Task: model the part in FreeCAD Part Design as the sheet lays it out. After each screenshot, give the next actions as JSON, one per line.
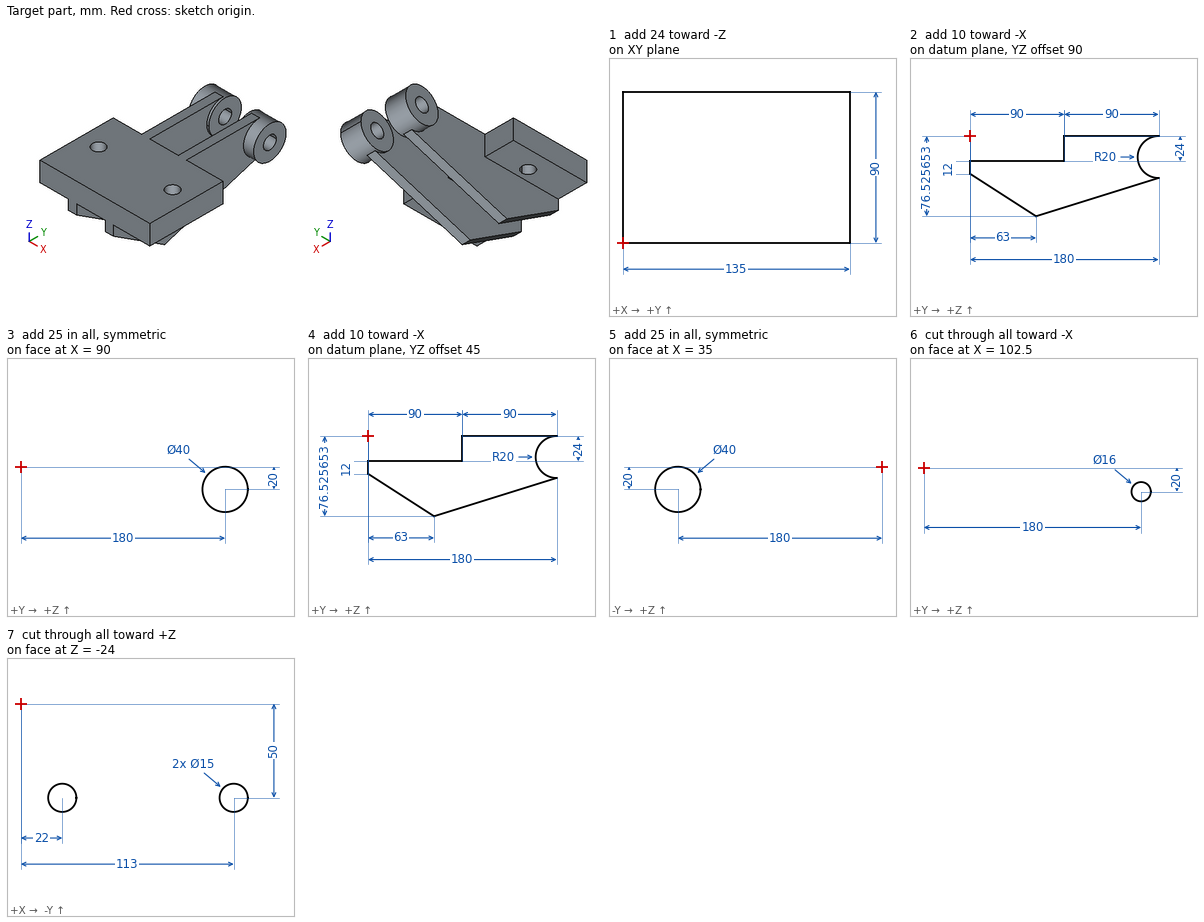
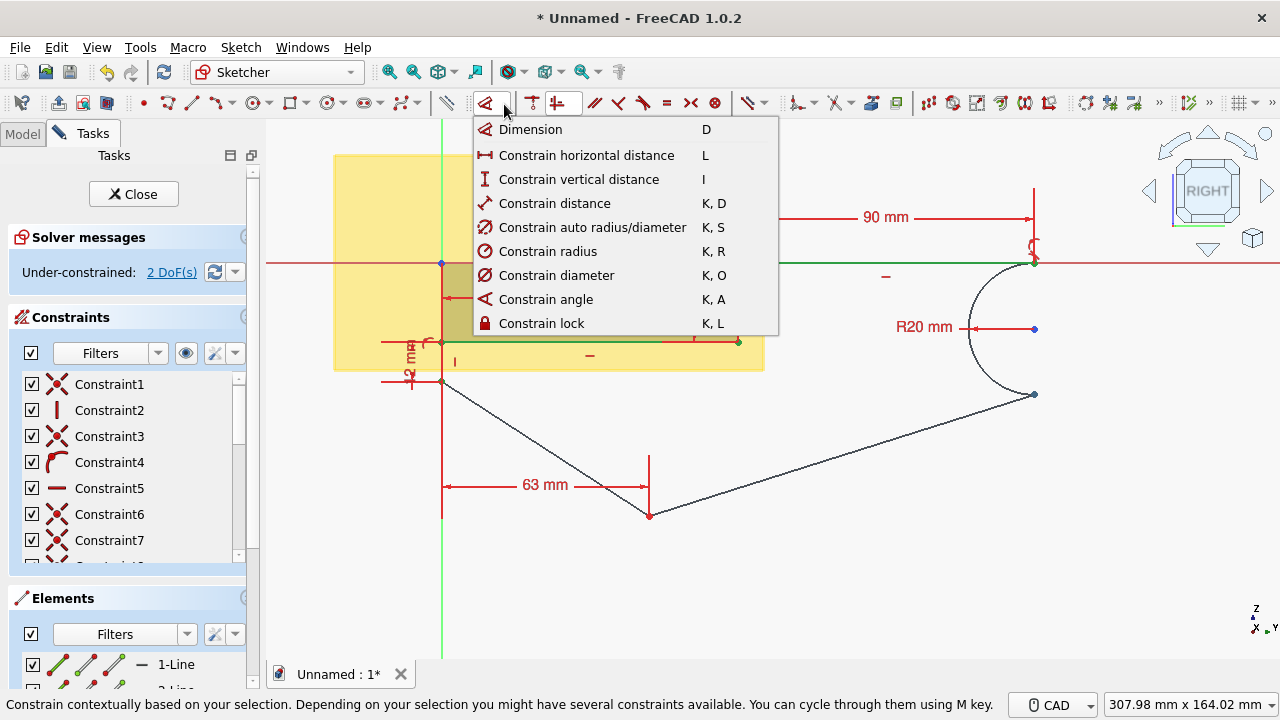
{"action": "left_click", "coordinate": [626, 155]}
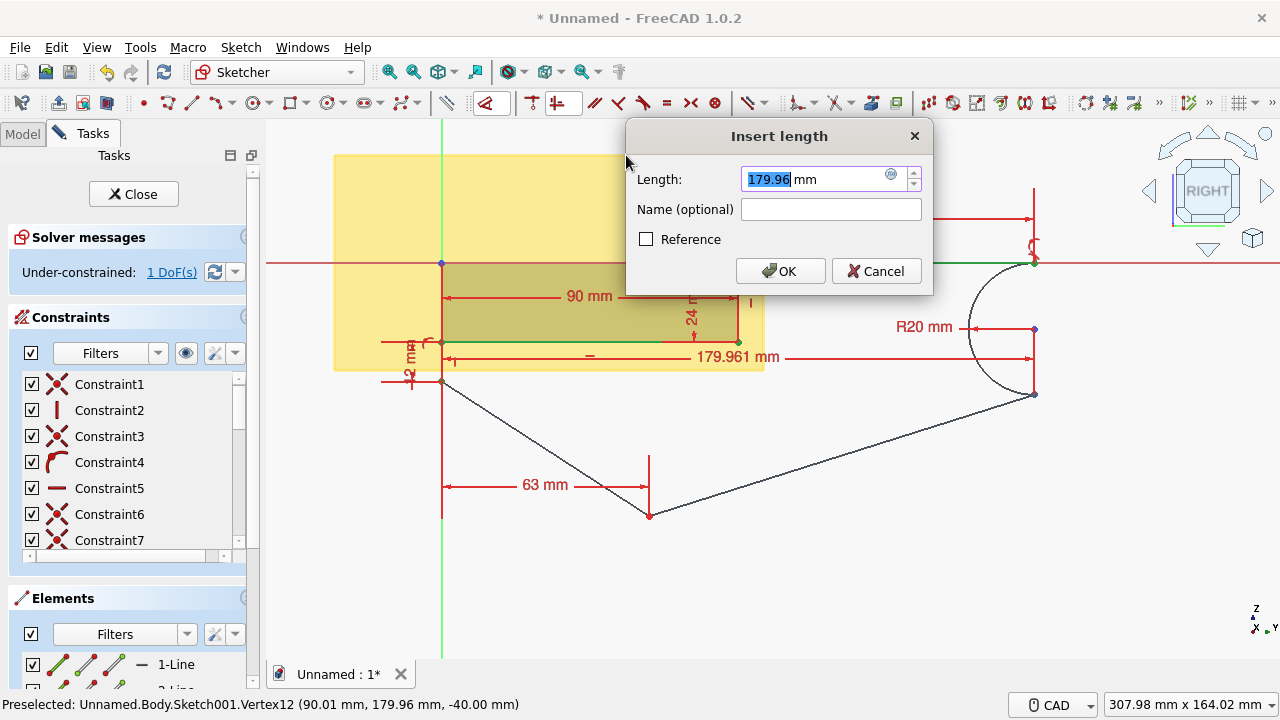
{"action": "type", "text": "180"}
{"action": "key", "text": "Return"}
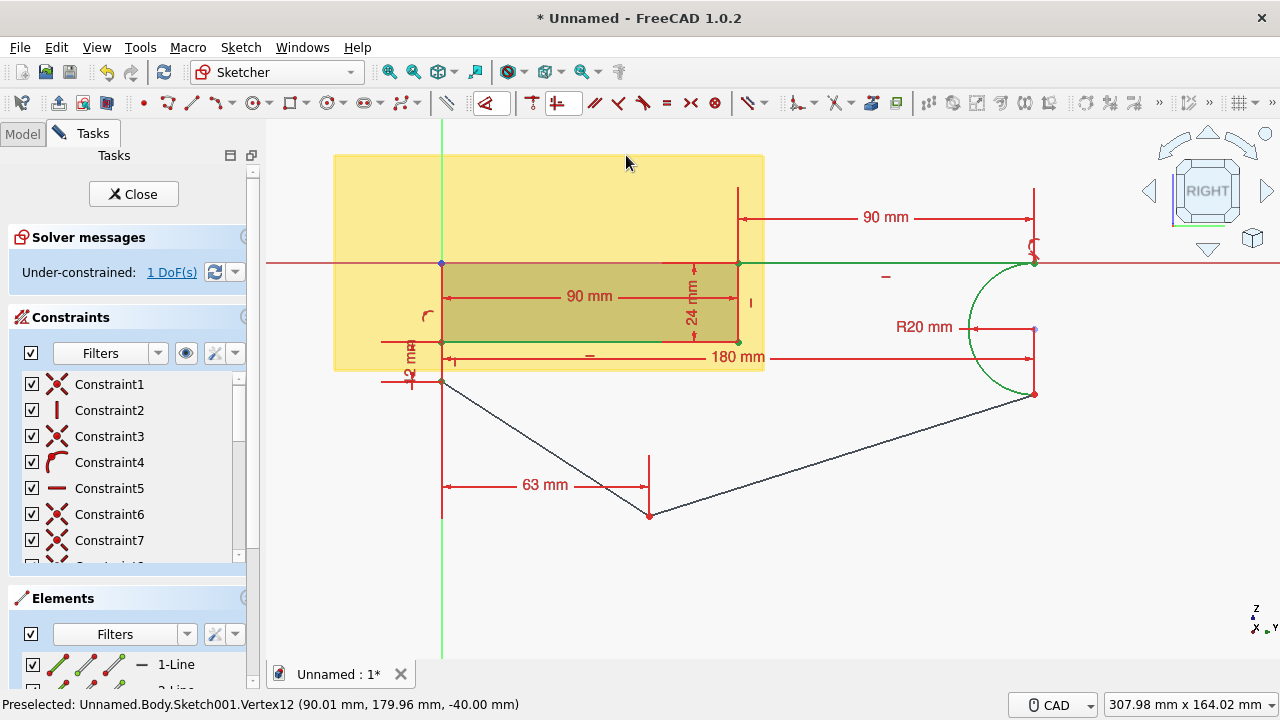
{"action": "left_click", "coordinate": [649, 516]}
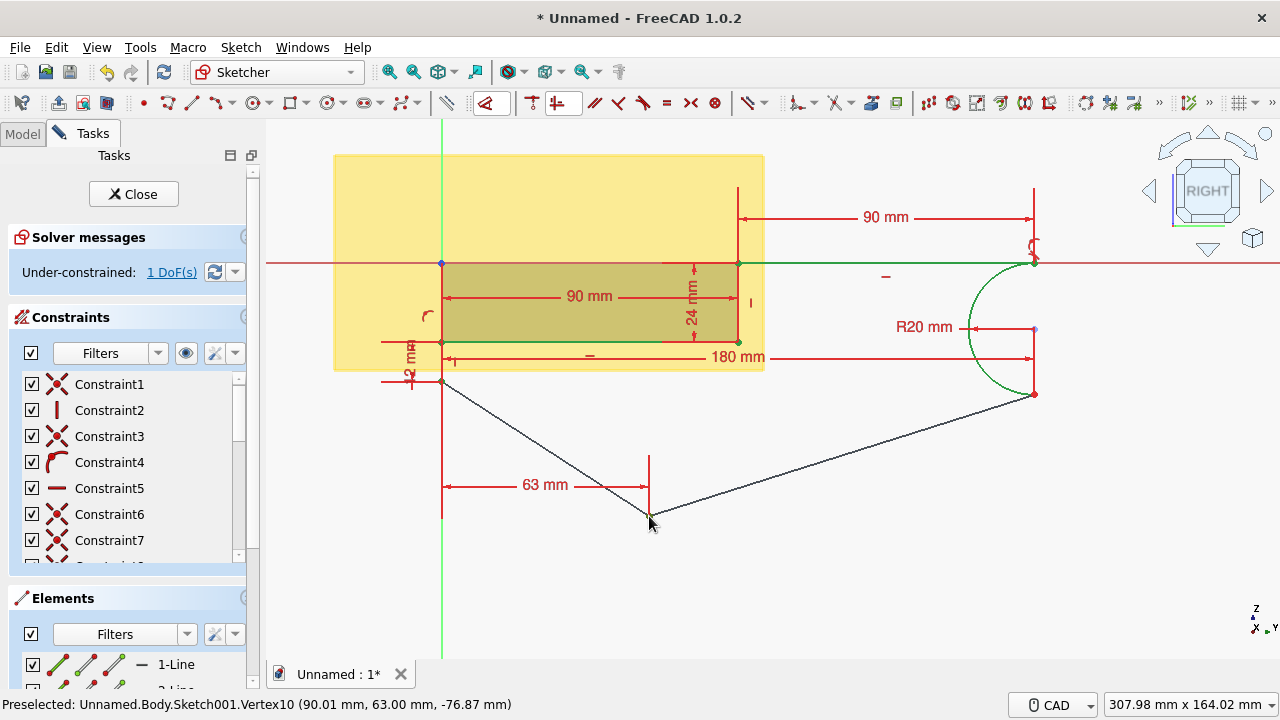
{"action": "left_click", "coordinate": [504, 104]}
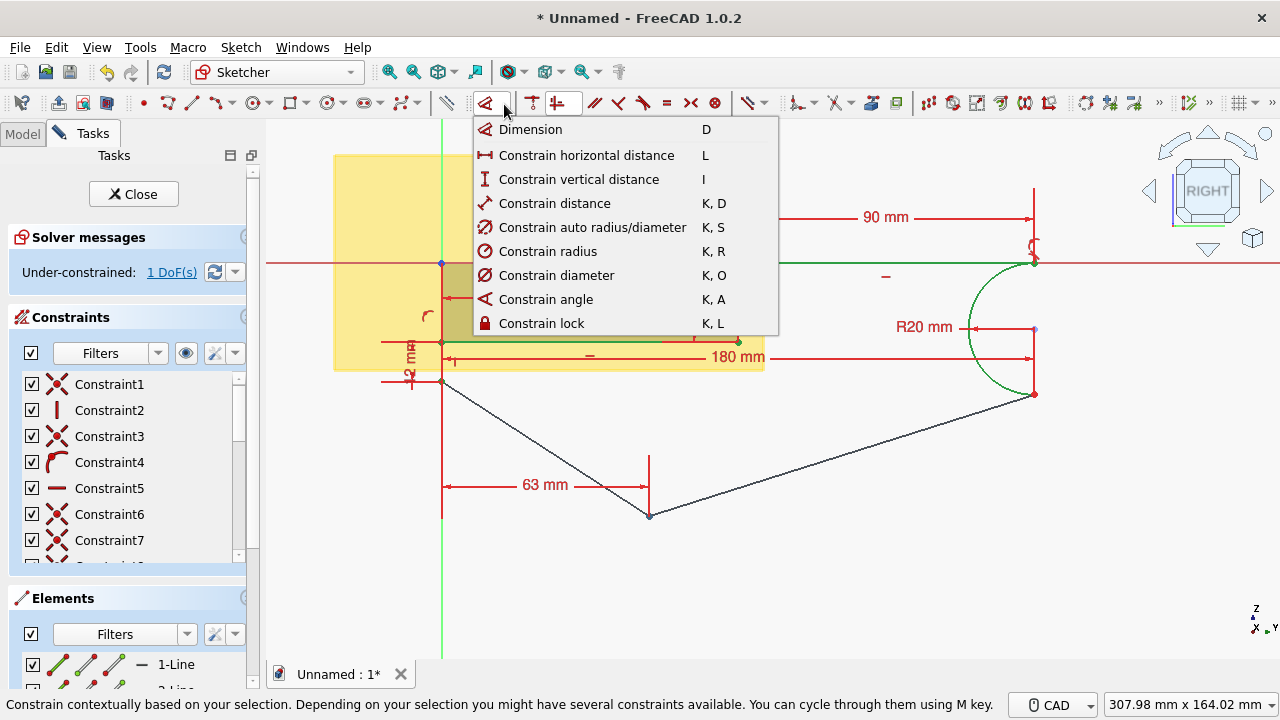
{"action": "left_click", "coordinate": [626, 179]}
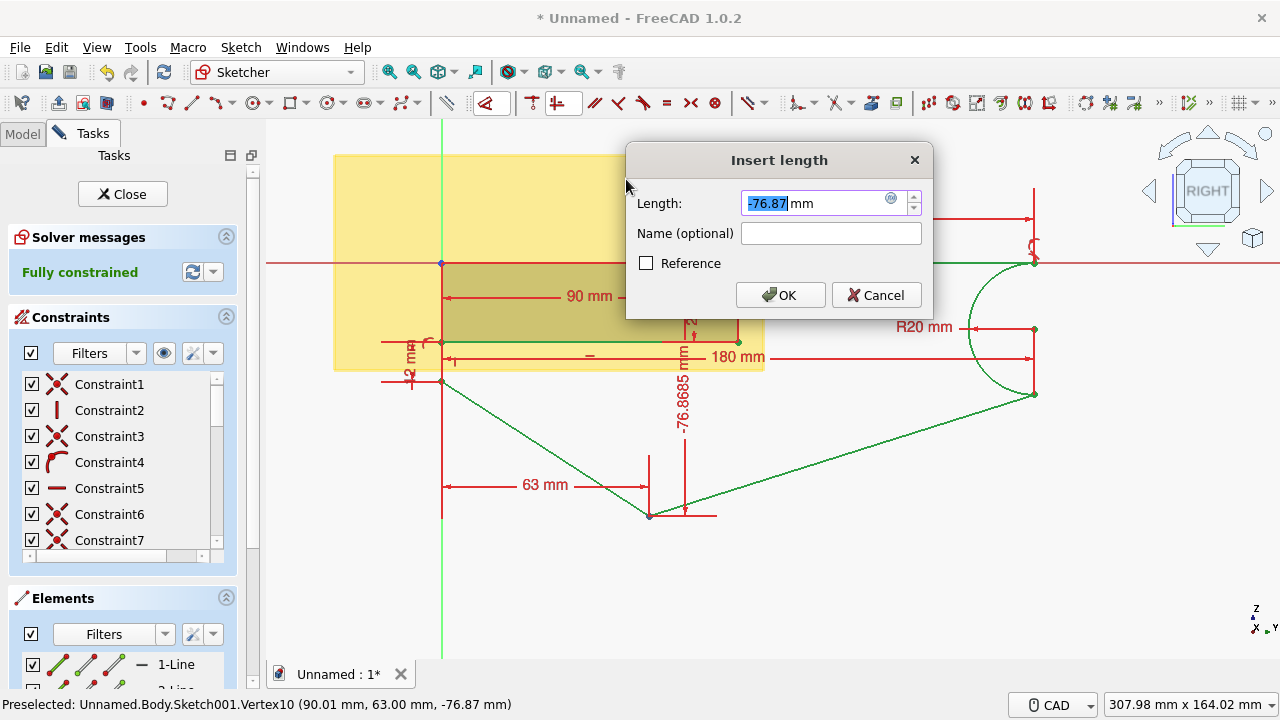
{"action": "type", "text": "-76.525653"}
{"action": "key", "text": "Return"}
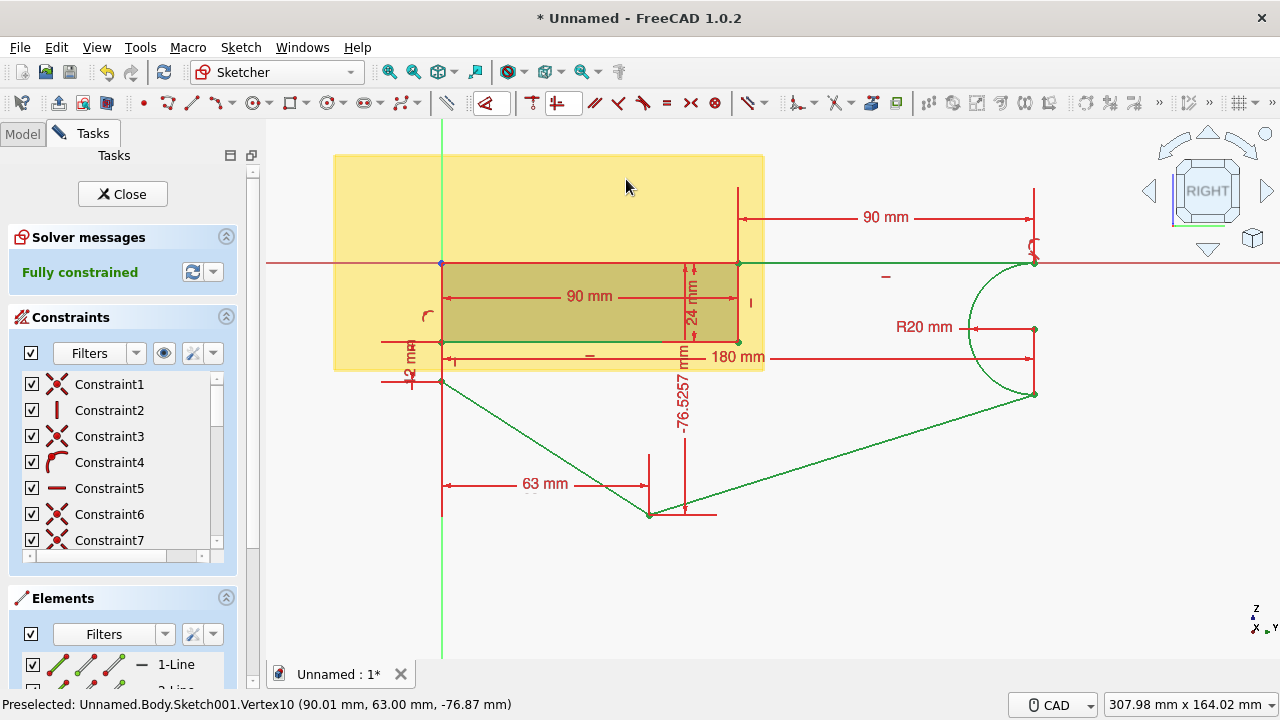
{"action": "left_click", "coordinate": [123, 194]}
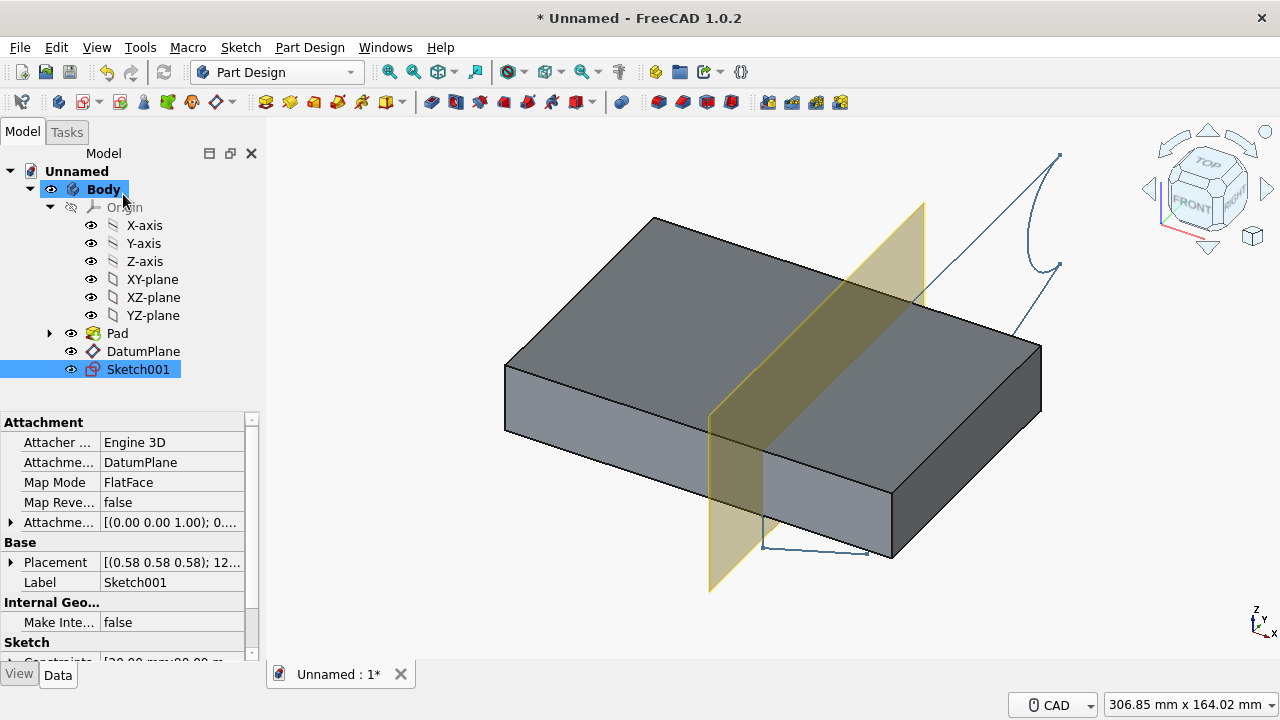
{"action": "left_click", "coordinate": [266, 102]}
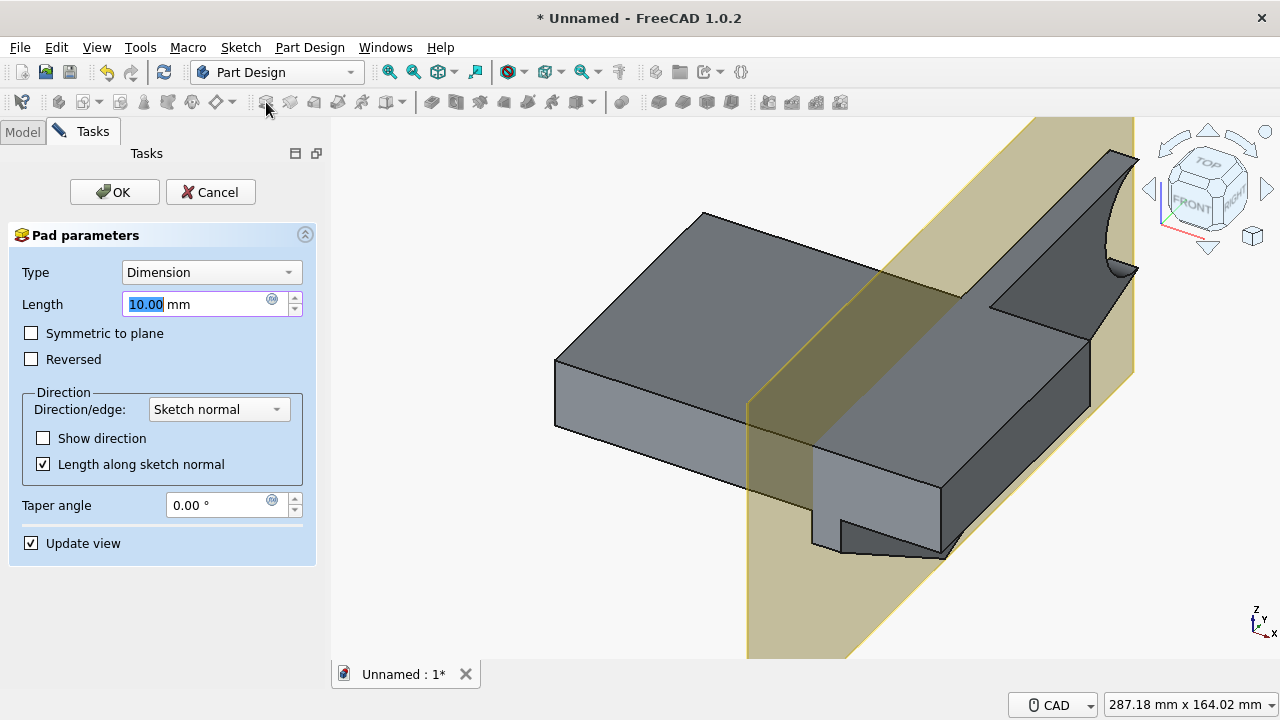
{"action": "type", "text": "10"}
{"action": "key", "text": "Tab"}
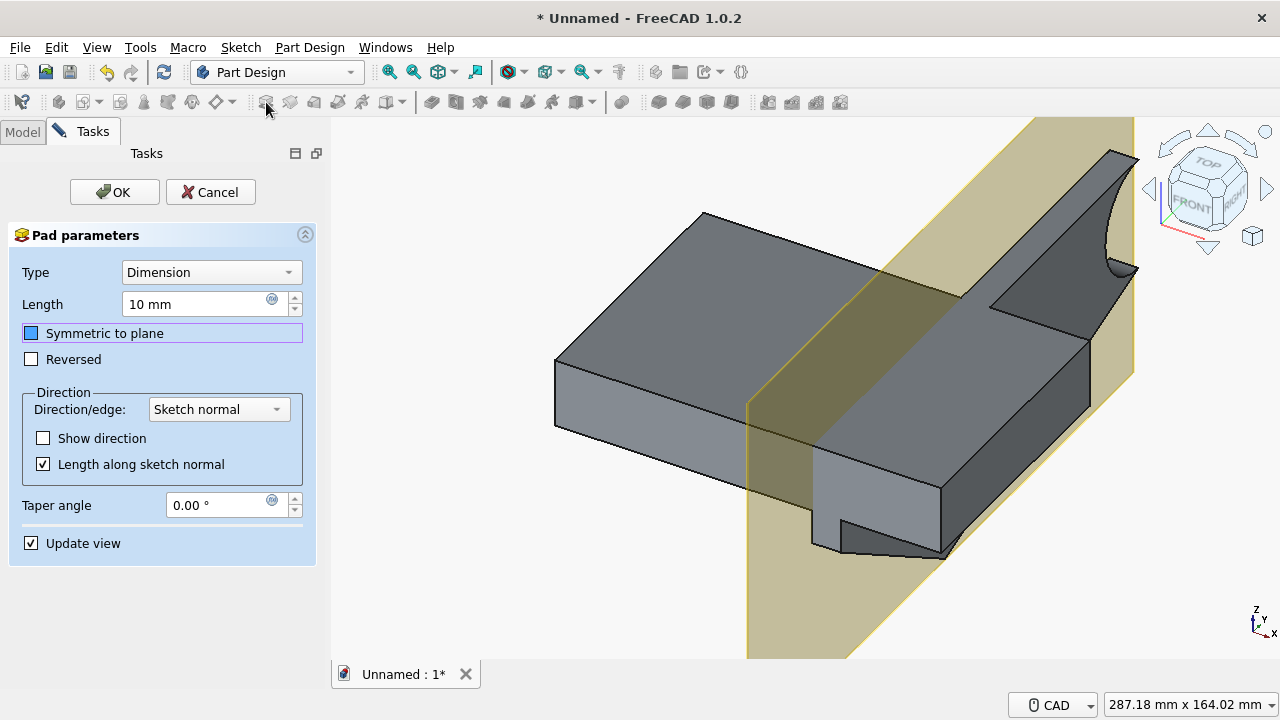
{"action": "left_click", "coordinate": [30, 359]}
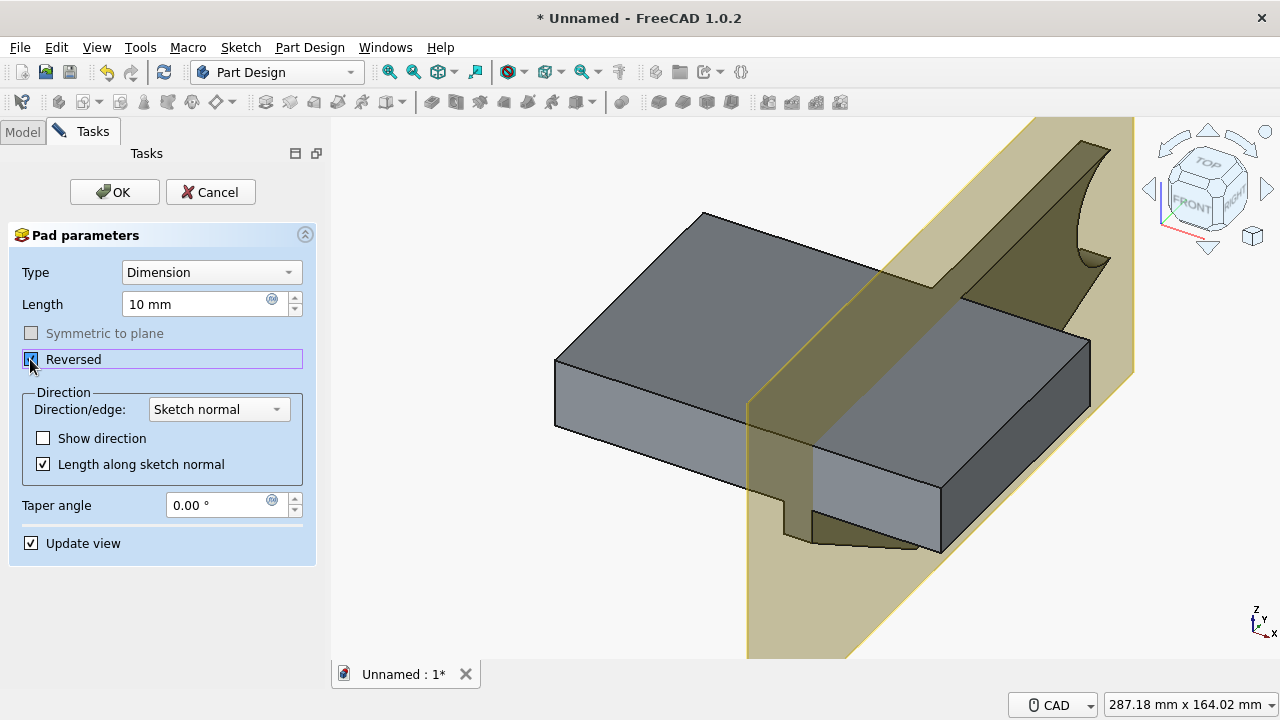
{"action": "left_click", "coordinate": [115, 192]}